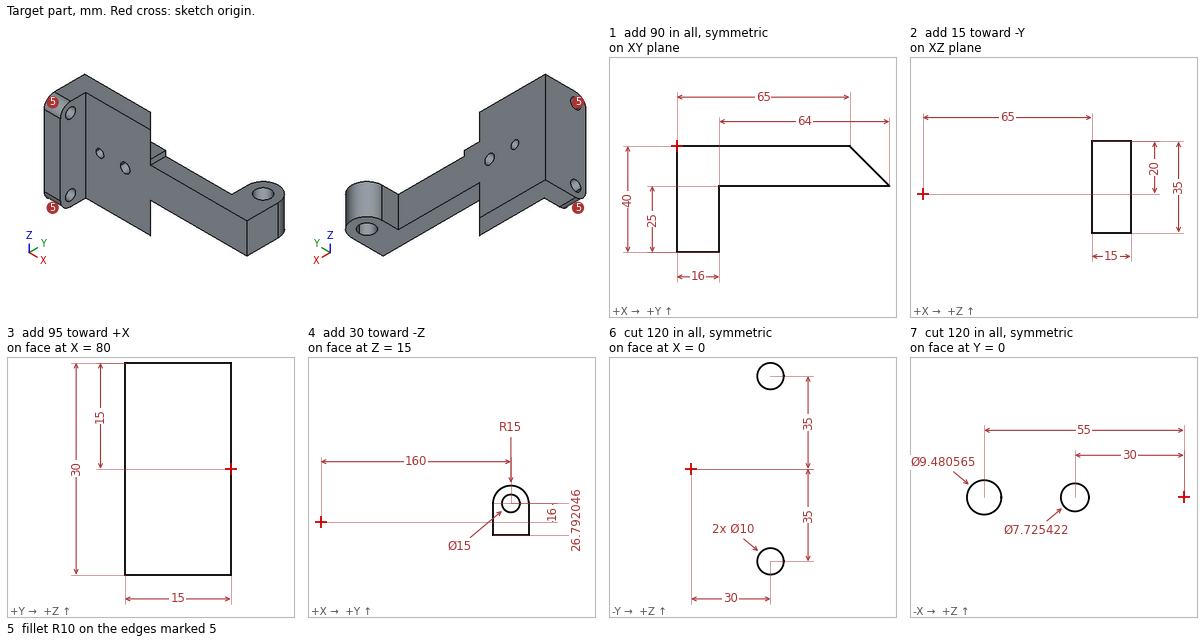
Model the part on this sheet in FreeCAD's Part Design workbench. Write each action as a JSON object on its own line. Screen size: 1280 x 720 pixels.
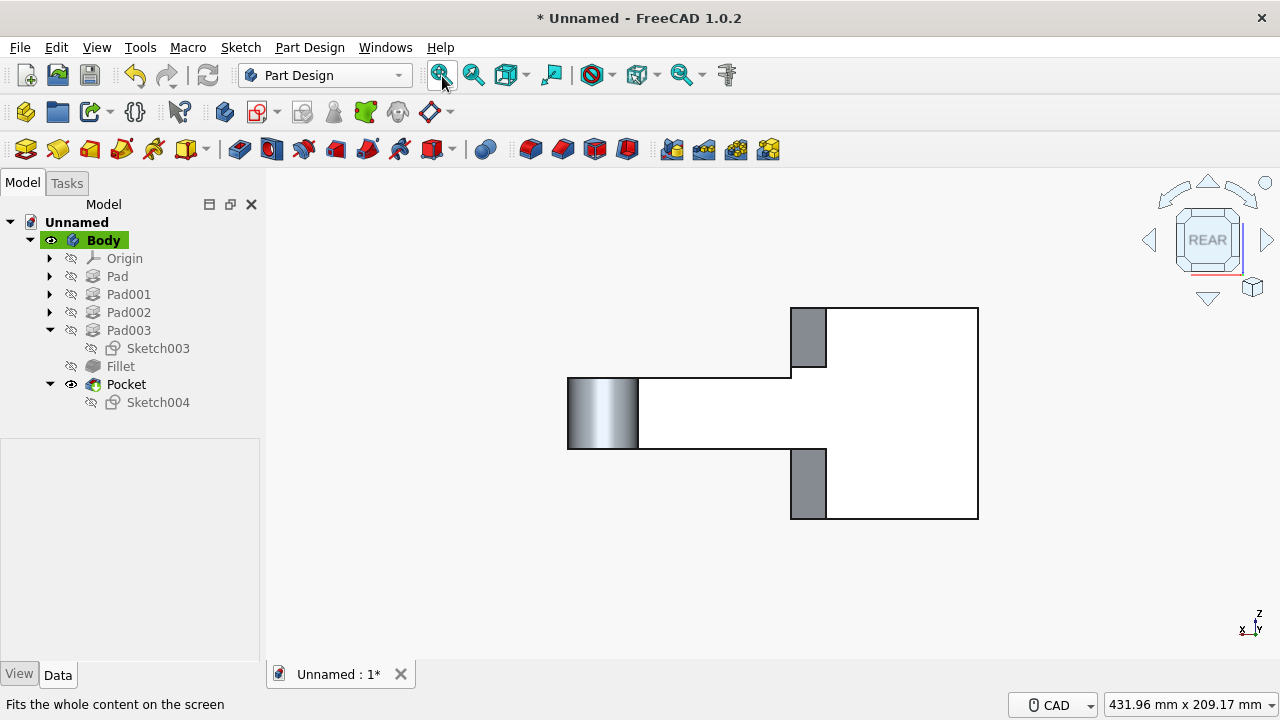
{"action": "left_click", "coordinate": [905, 382]}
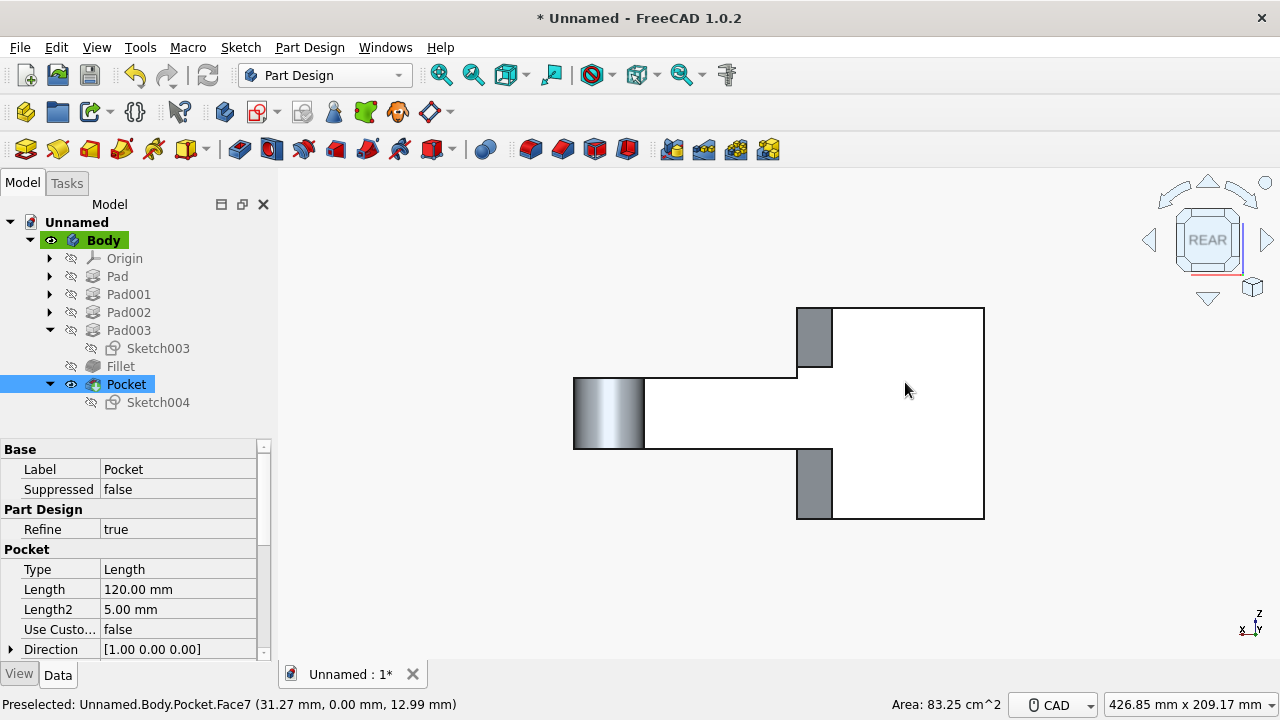
{"action": "left_click", "coordinate": [258, 112]}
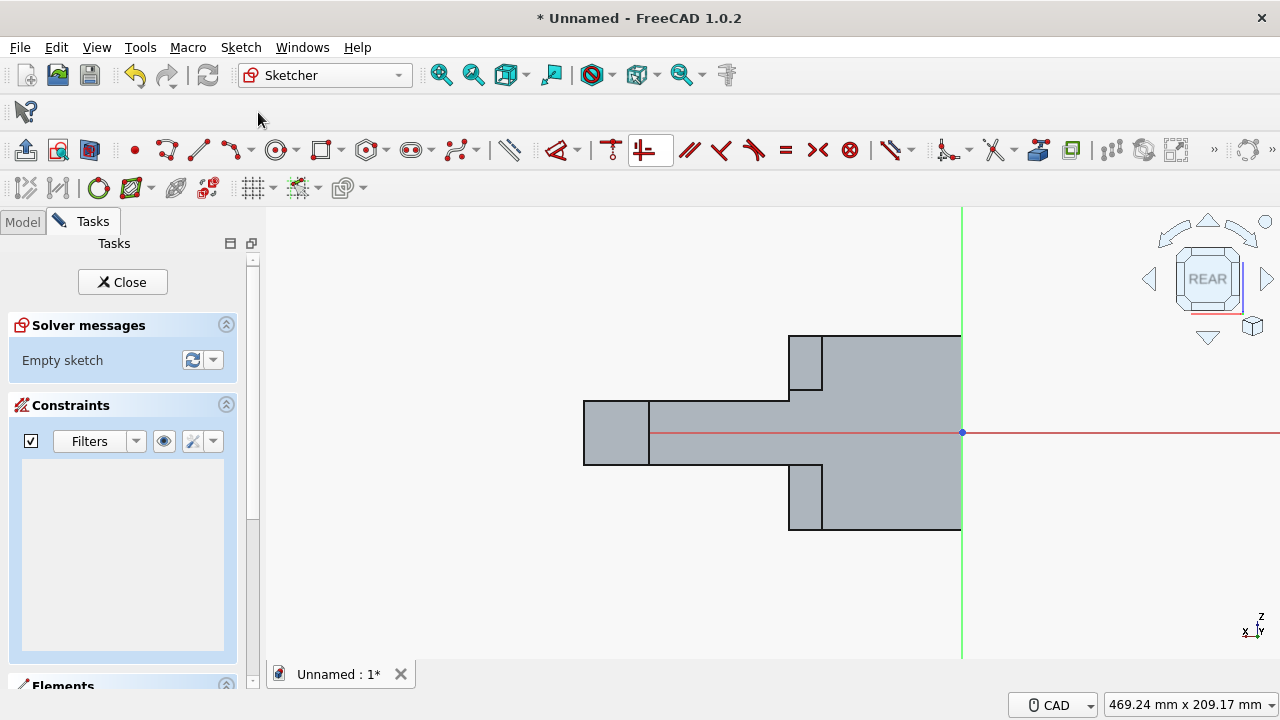
{"action": "scroll", "coordinate": [946, 433], "scroll_direction": "up", "scroll_amount": 8}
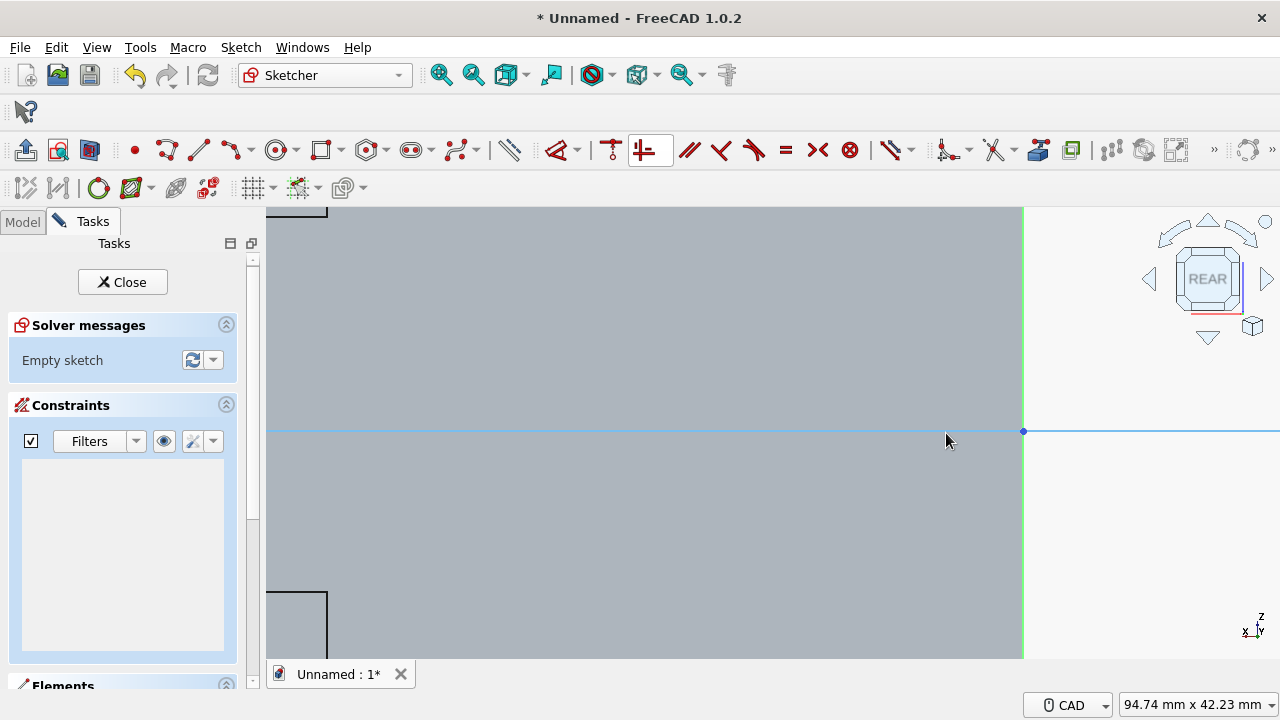
{"action": "left_click", "coordinate": [276, 150]}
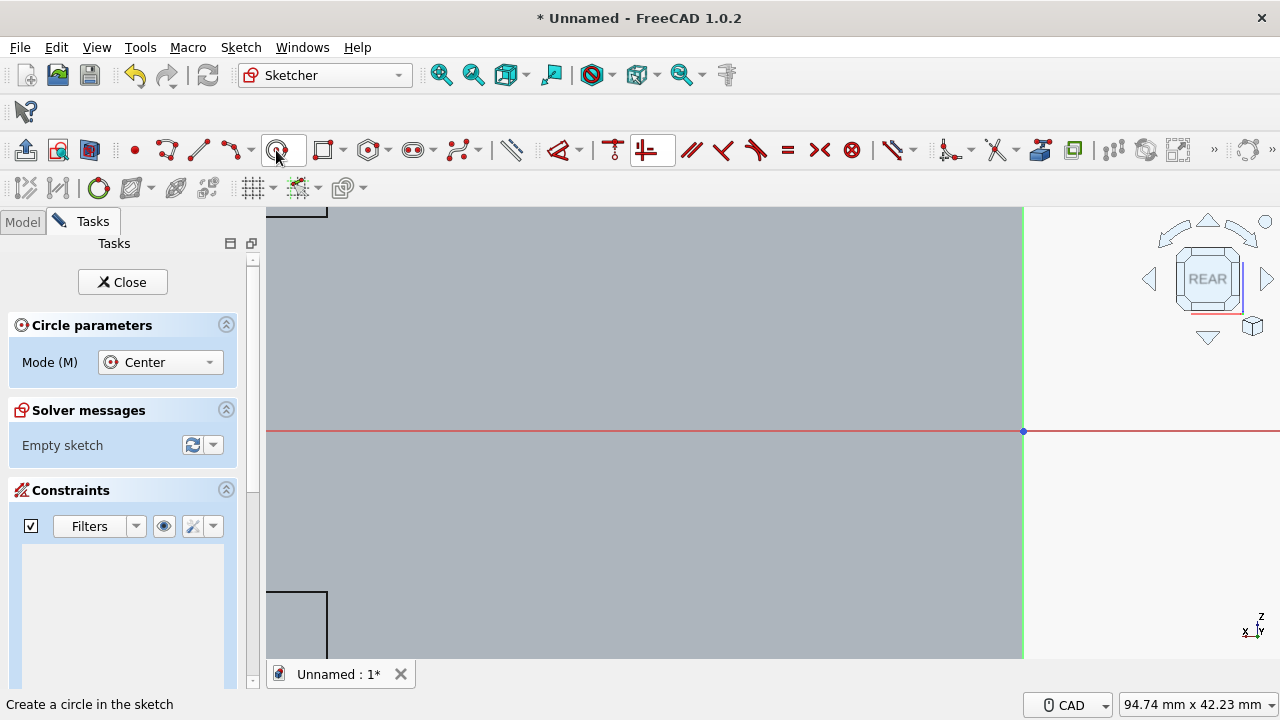
{"action": "left_click", "coordinate": [702, 431]}
{"action": "mouse_move", "coordinate": [731, 402]}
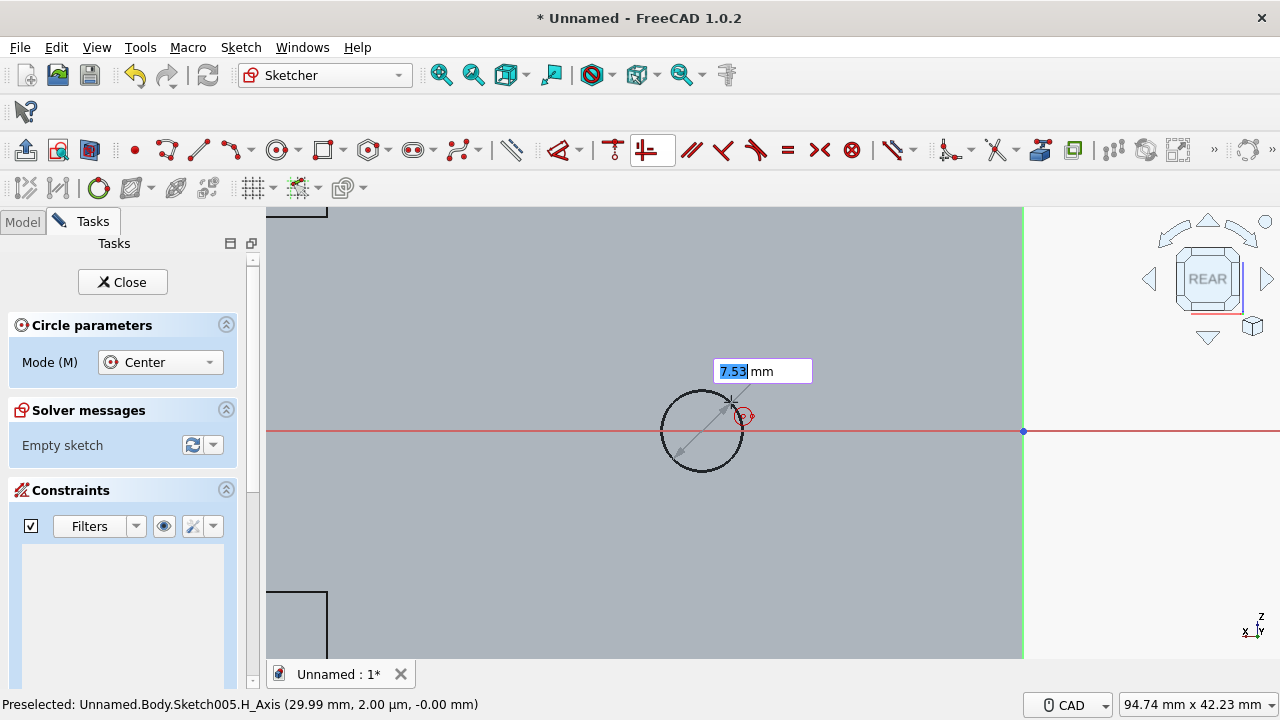
{"action": "type", "text": "7.725422"}
{"action": "key", "text": "Return"}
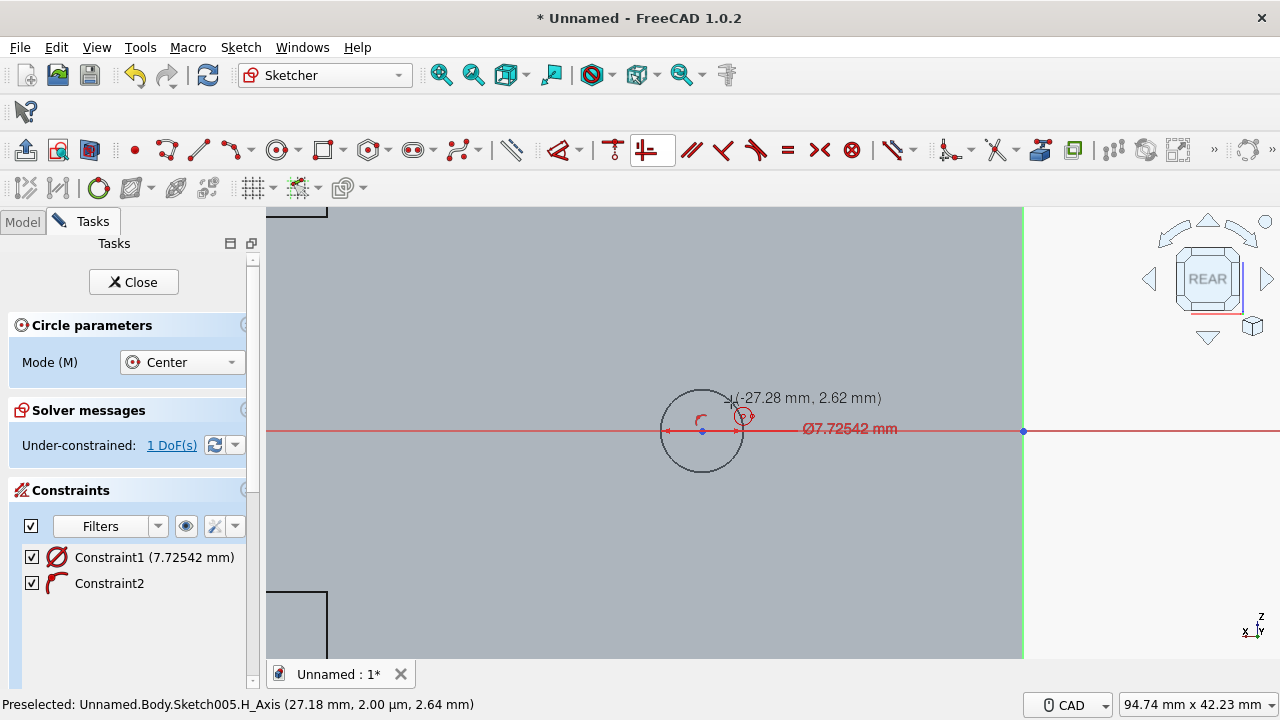
{"action": "left_click", "coordinate": [434, 431]}
{"action": "mouse_move", "coordinate": [470, 395]}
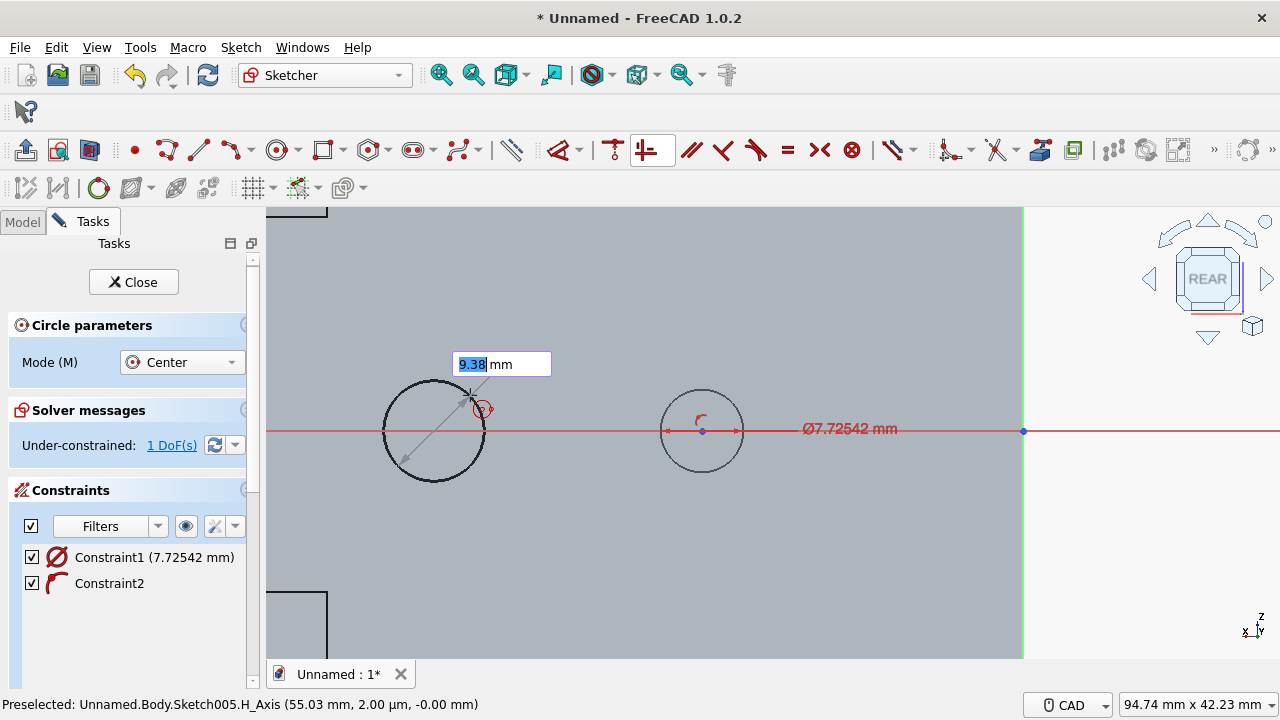
{"action": "type", "text": "9.480565"}
{"action": "key", "text": "Return"}
{"action": "key", "text": "Escape"}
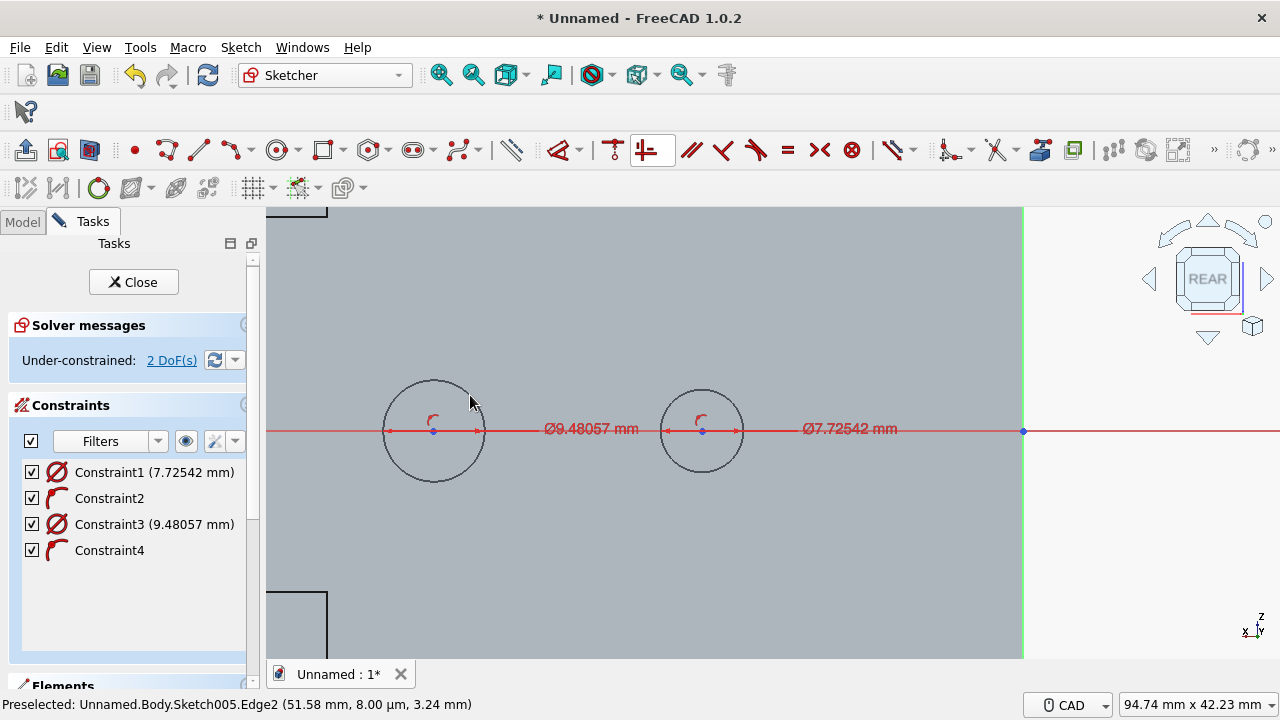
{"action": "key", "text": "d"}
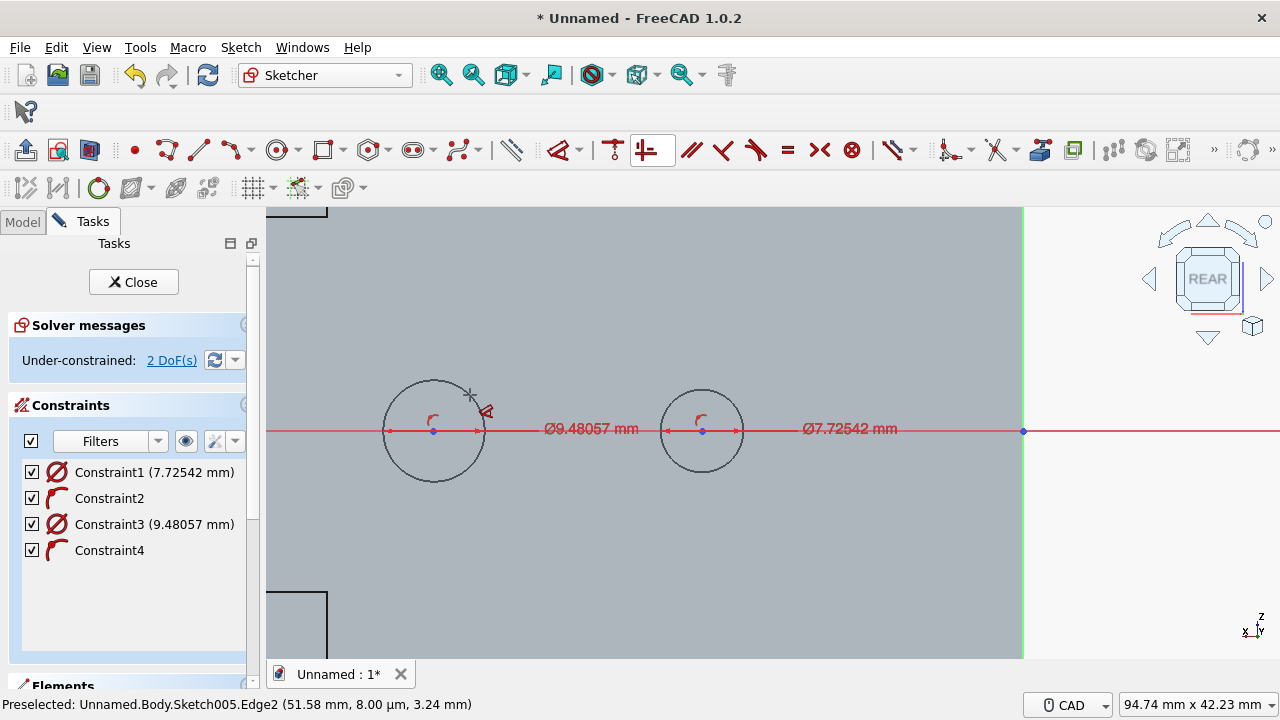
{"action": "left_click", "coordinate": [702, 431]}
{"action": "left_click", "coordinate": [863, 465]}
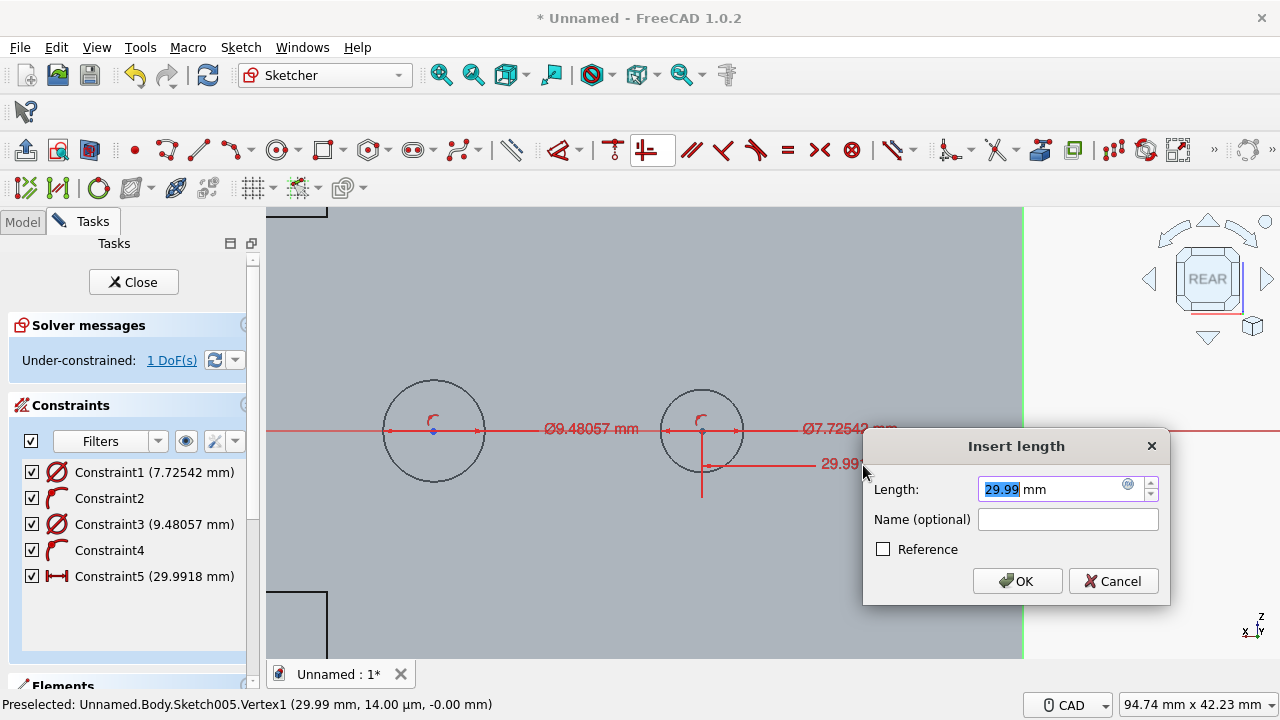
{"action": "type", "text": "30"}
{"action": "key", "text": "Return"}